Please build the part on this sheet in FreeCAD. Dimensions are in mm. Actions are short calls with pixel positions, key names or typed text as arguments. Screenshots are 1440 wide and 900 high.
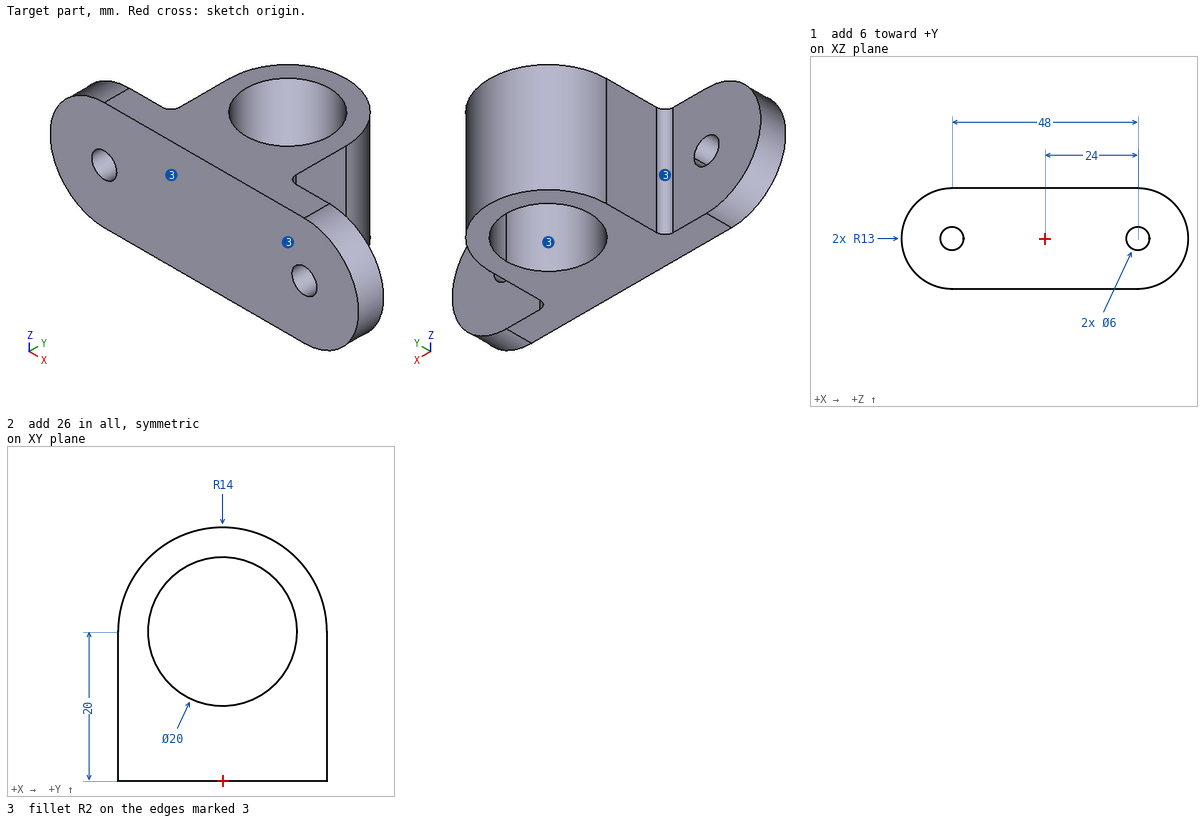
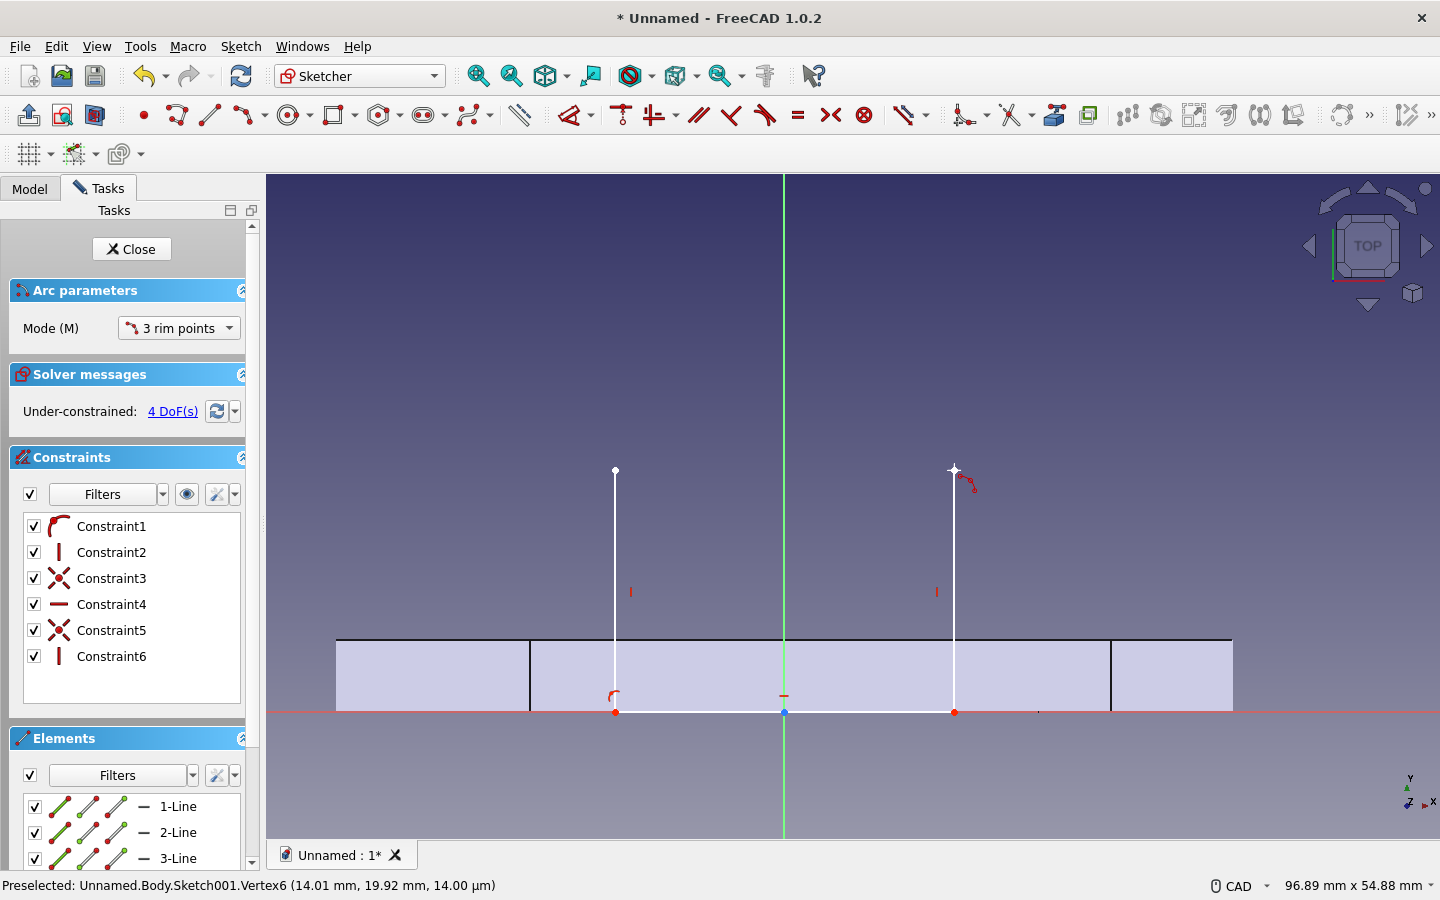
click(954, 471)
click(615, 471)
click(837, 309)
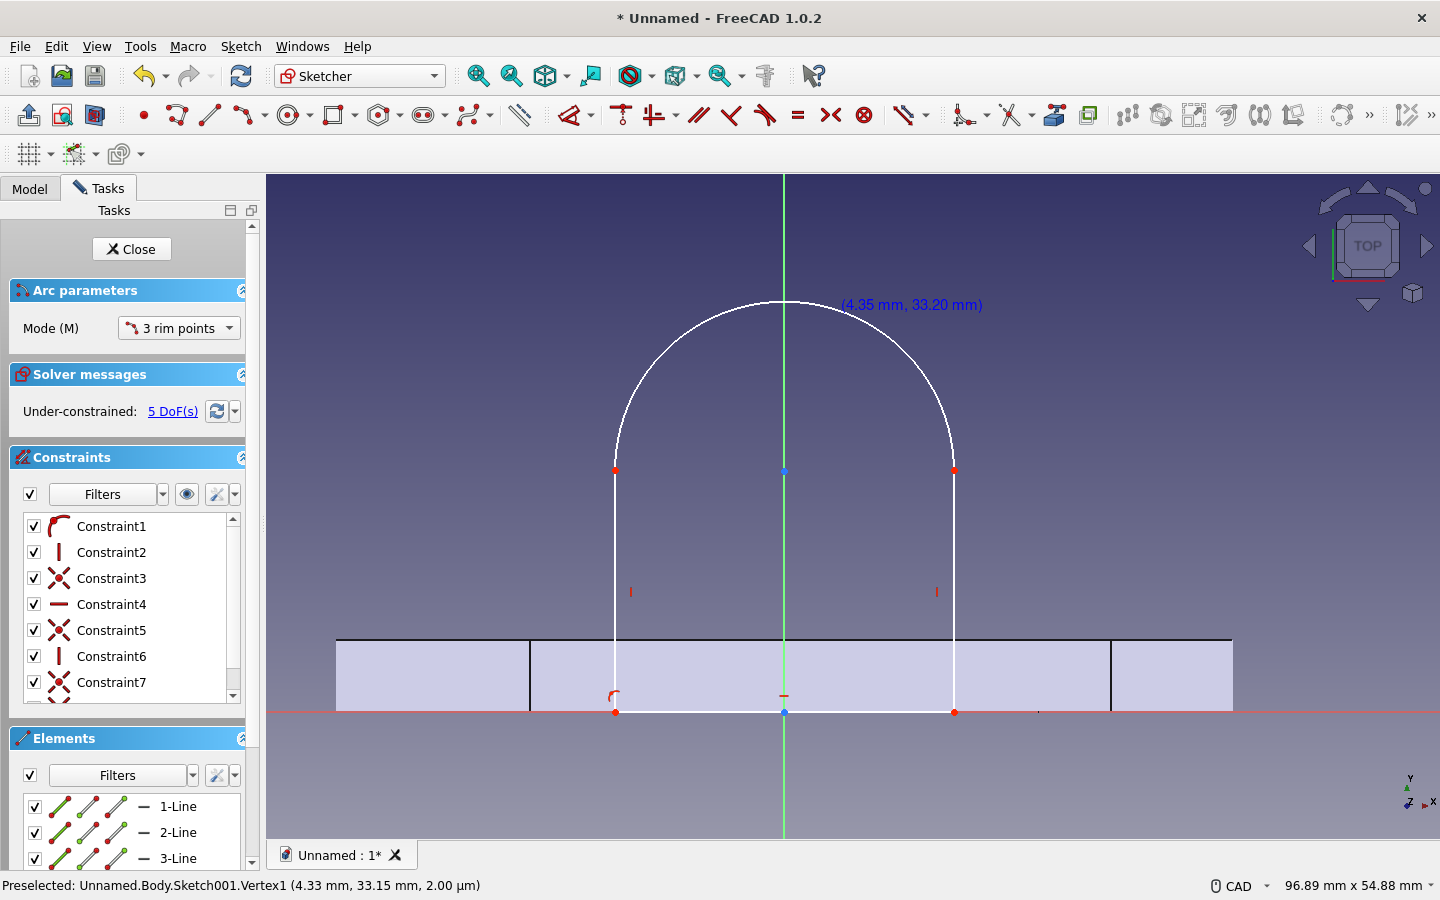
key(g)
key(c)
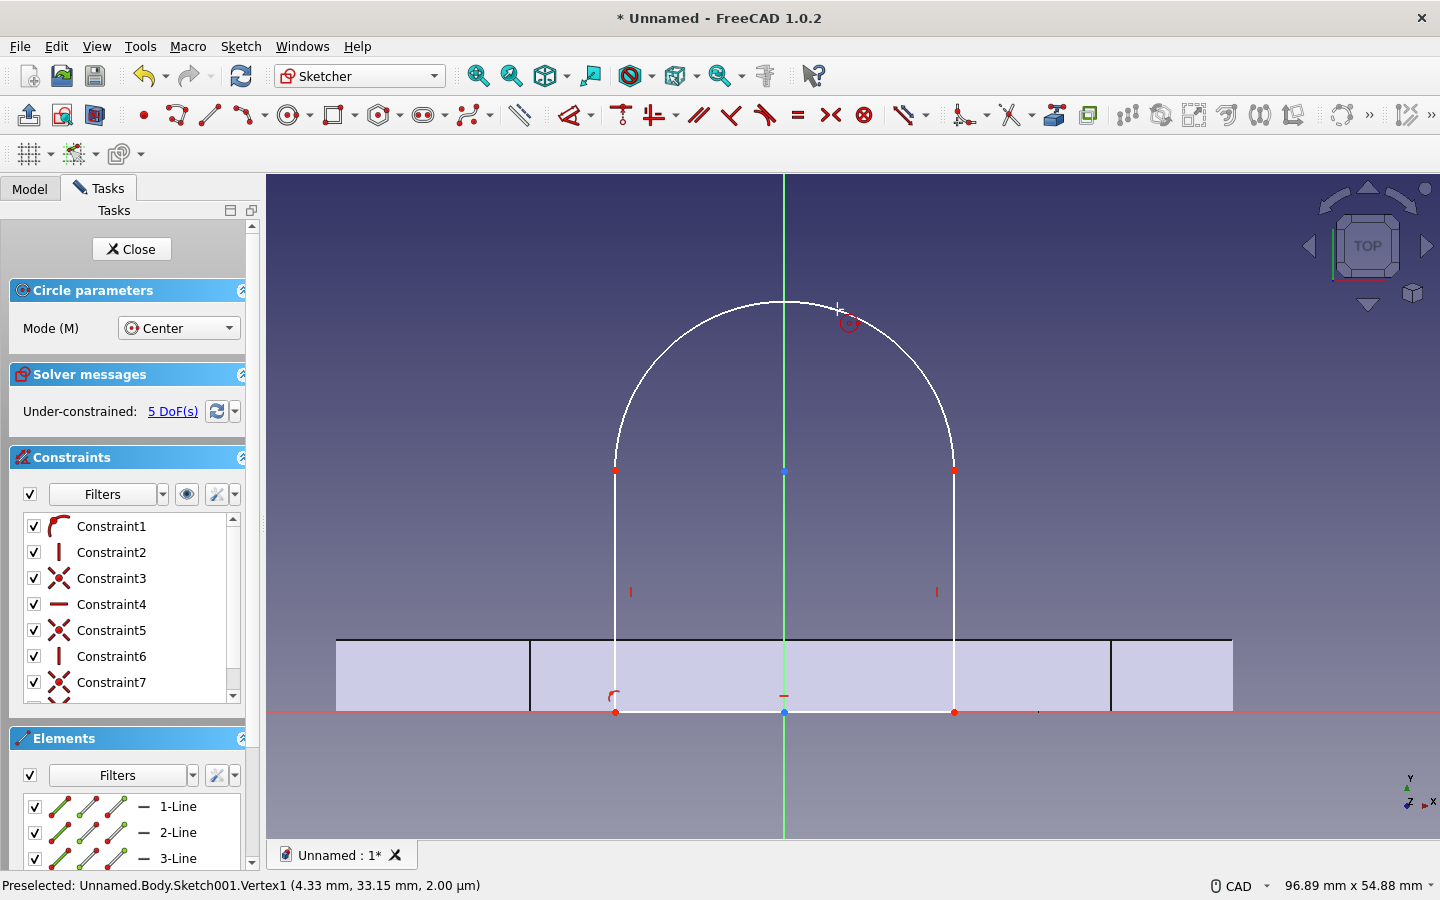
click(784, 470)
click(870, 384)
key(Escape)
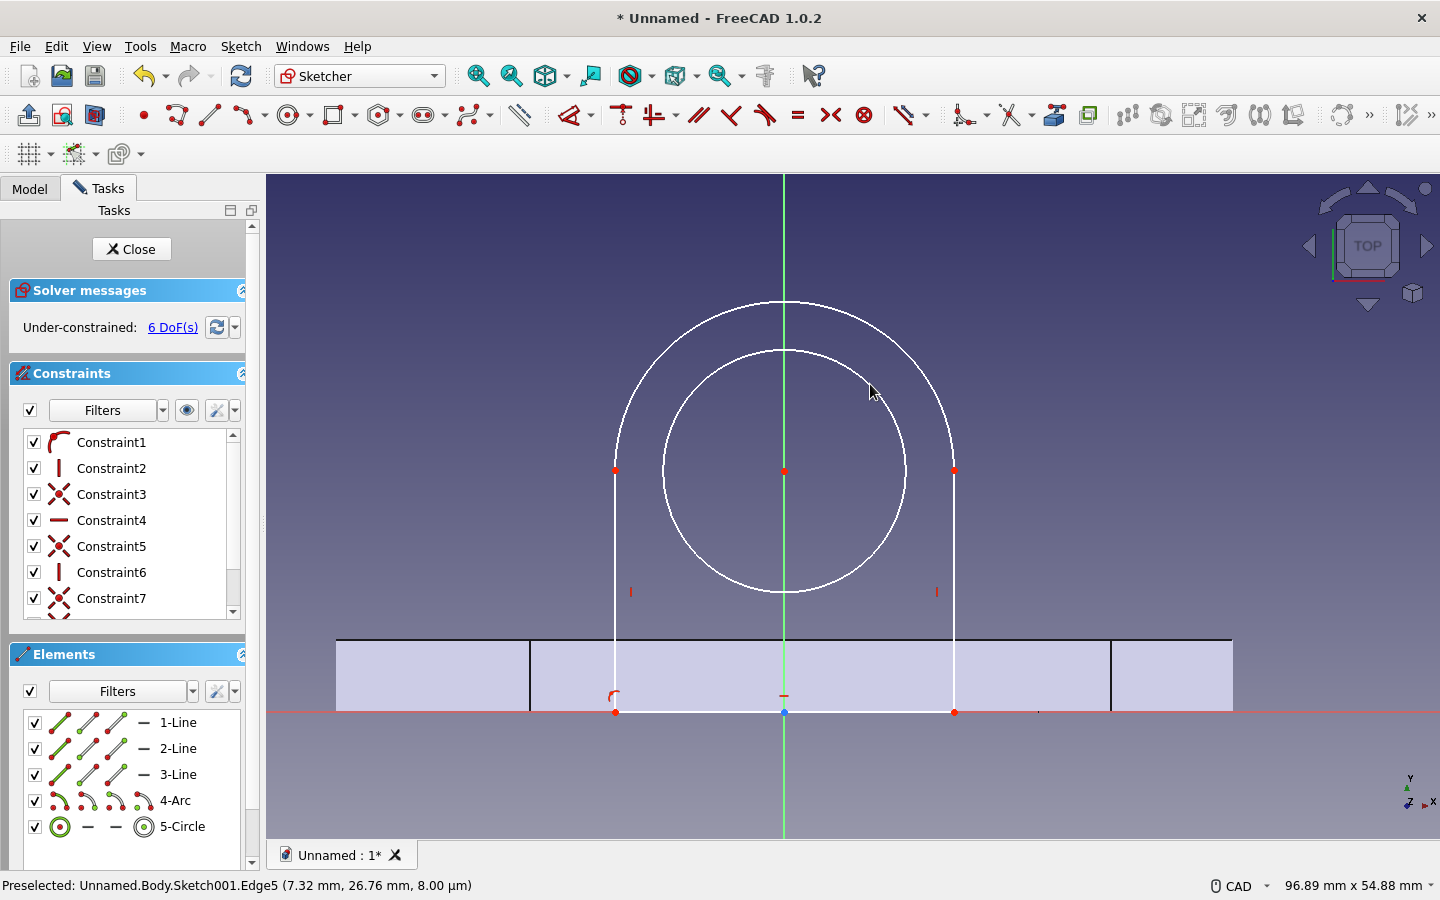
click(615, 543)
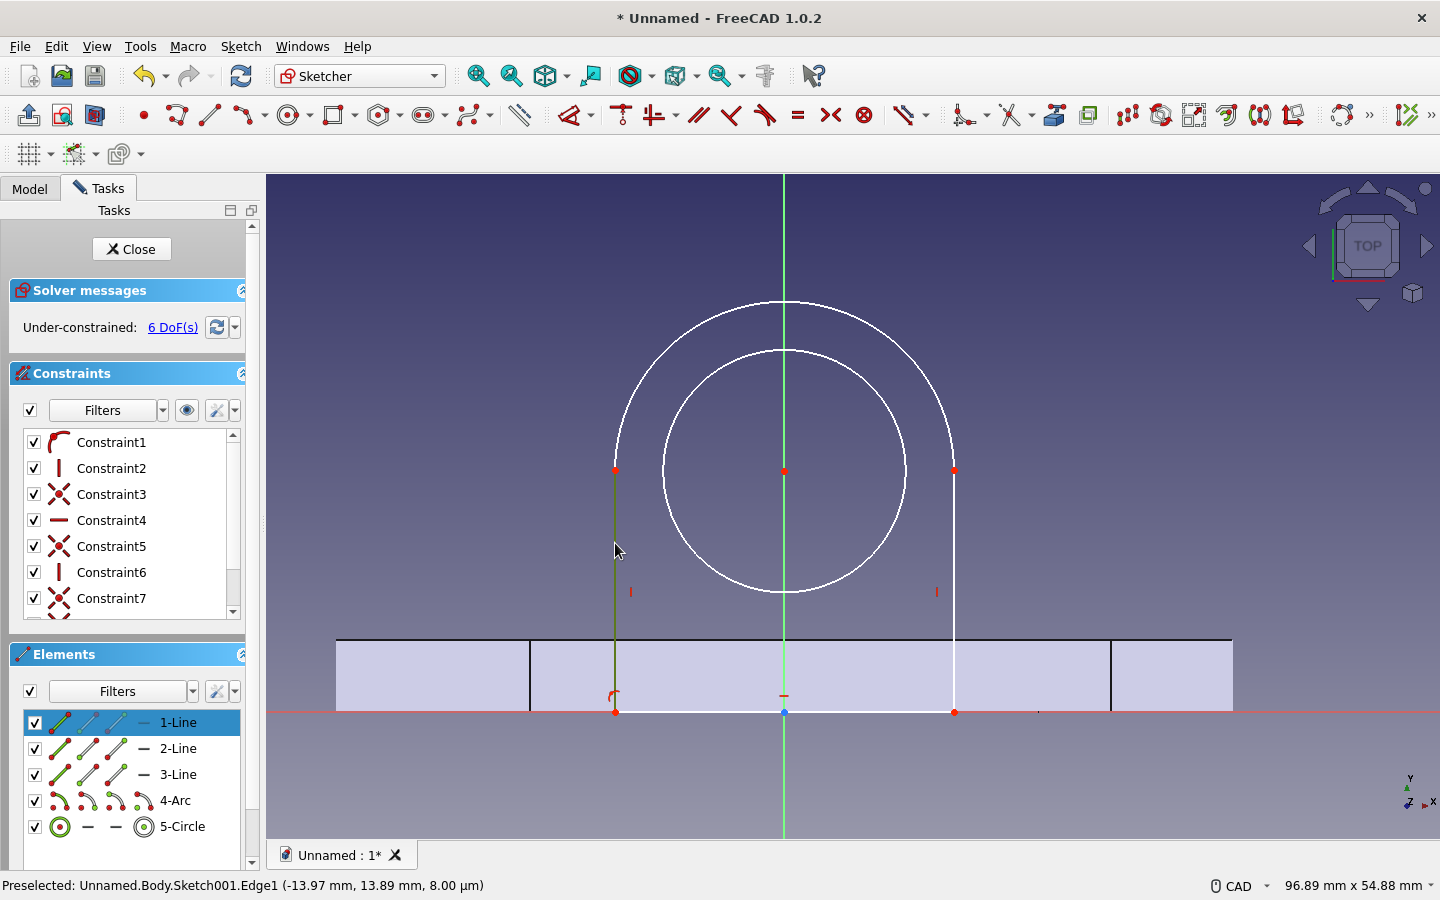
click(884, 334)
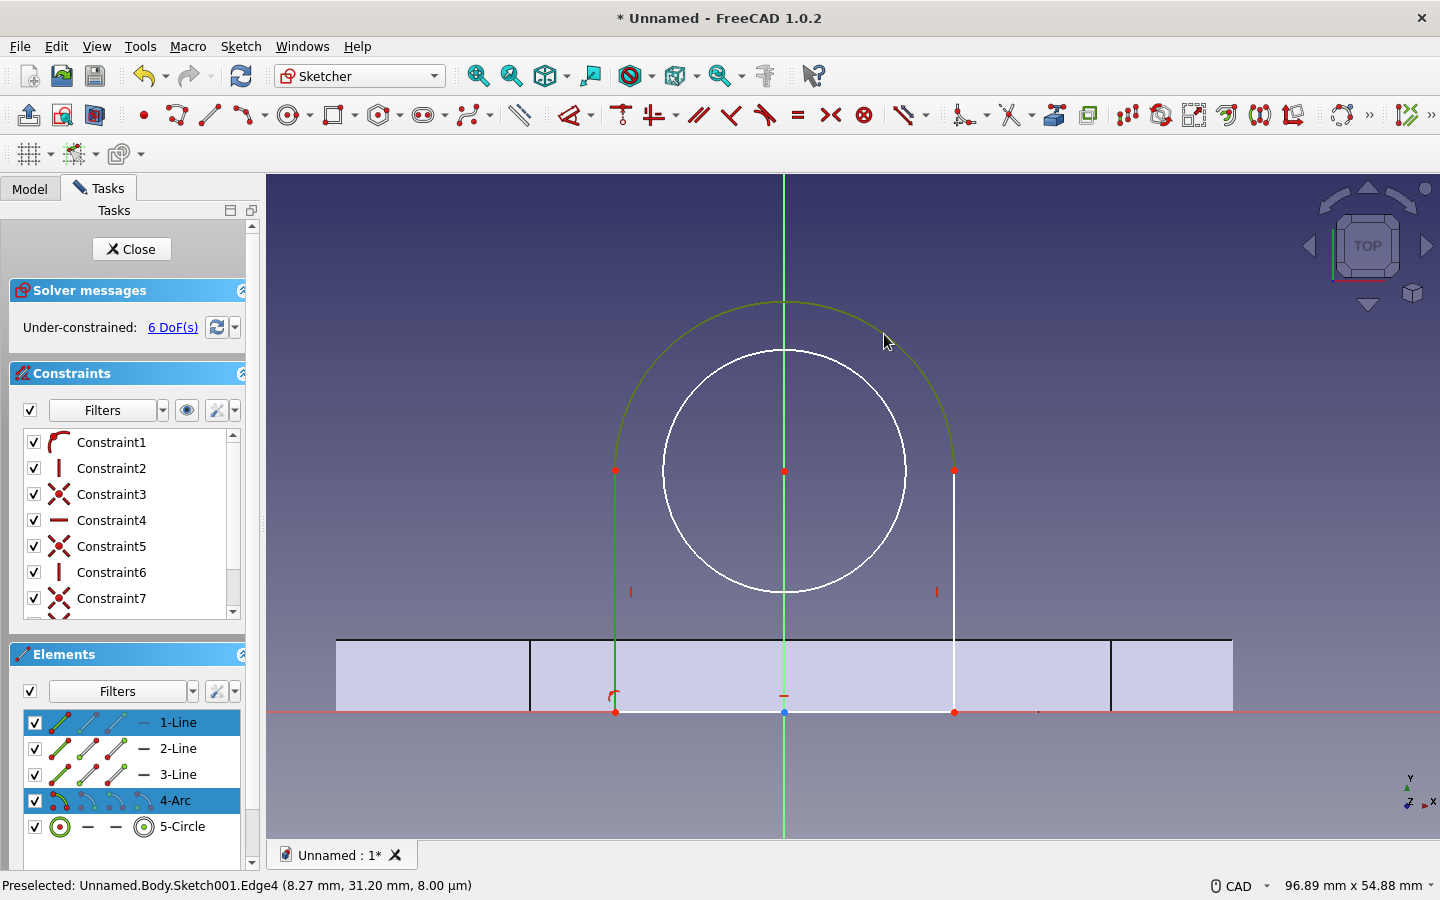
click(765, 116)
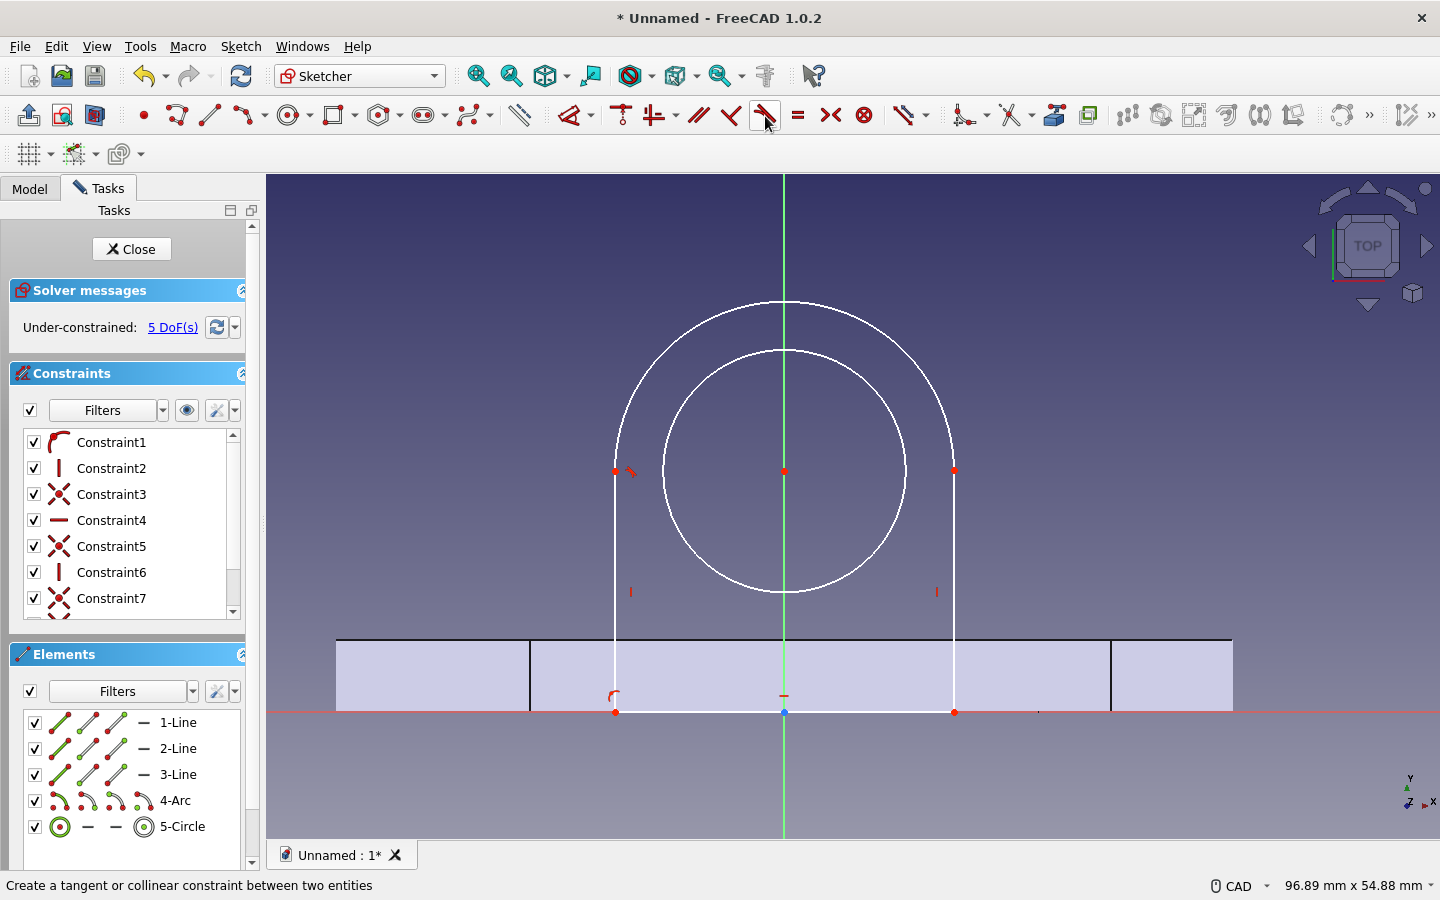
click(954, 640)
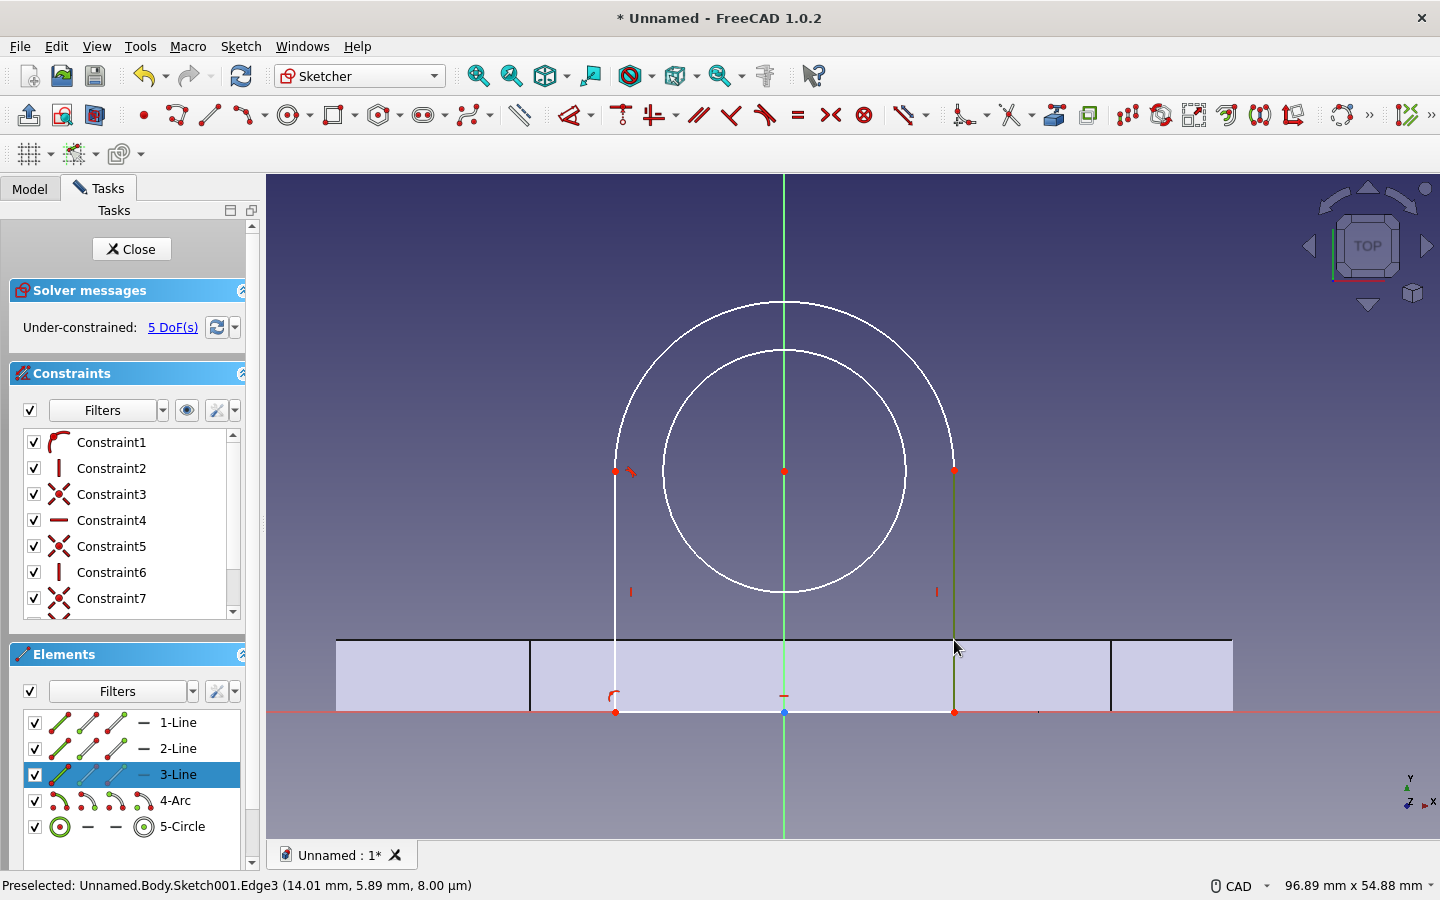
click(884, 334)